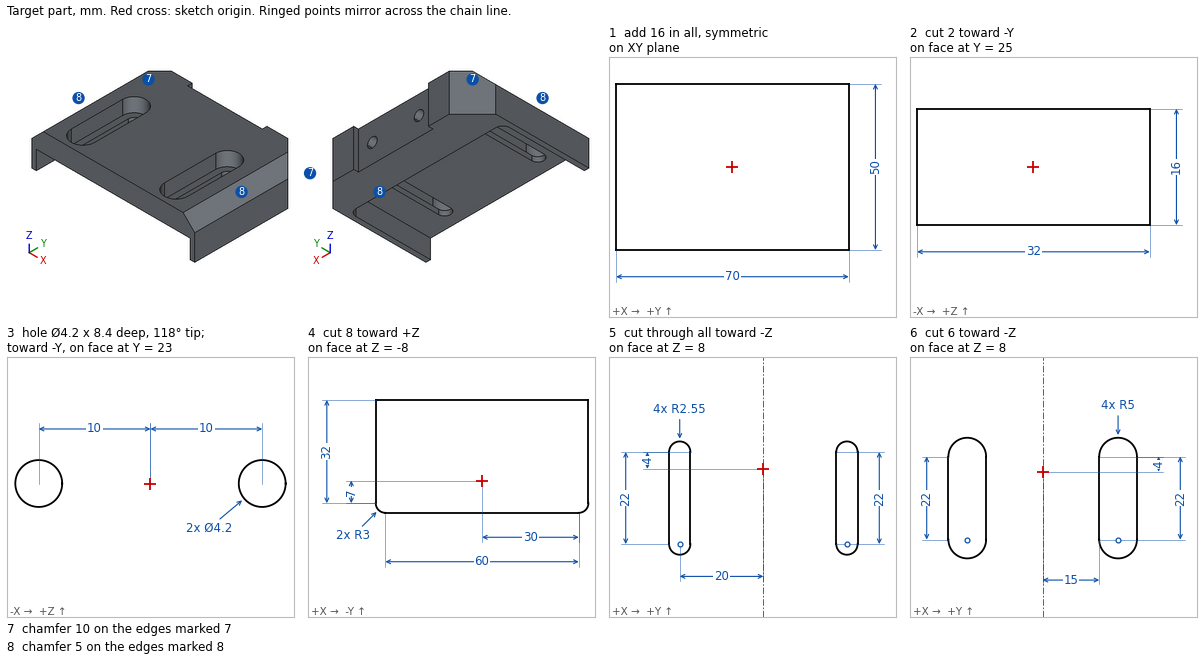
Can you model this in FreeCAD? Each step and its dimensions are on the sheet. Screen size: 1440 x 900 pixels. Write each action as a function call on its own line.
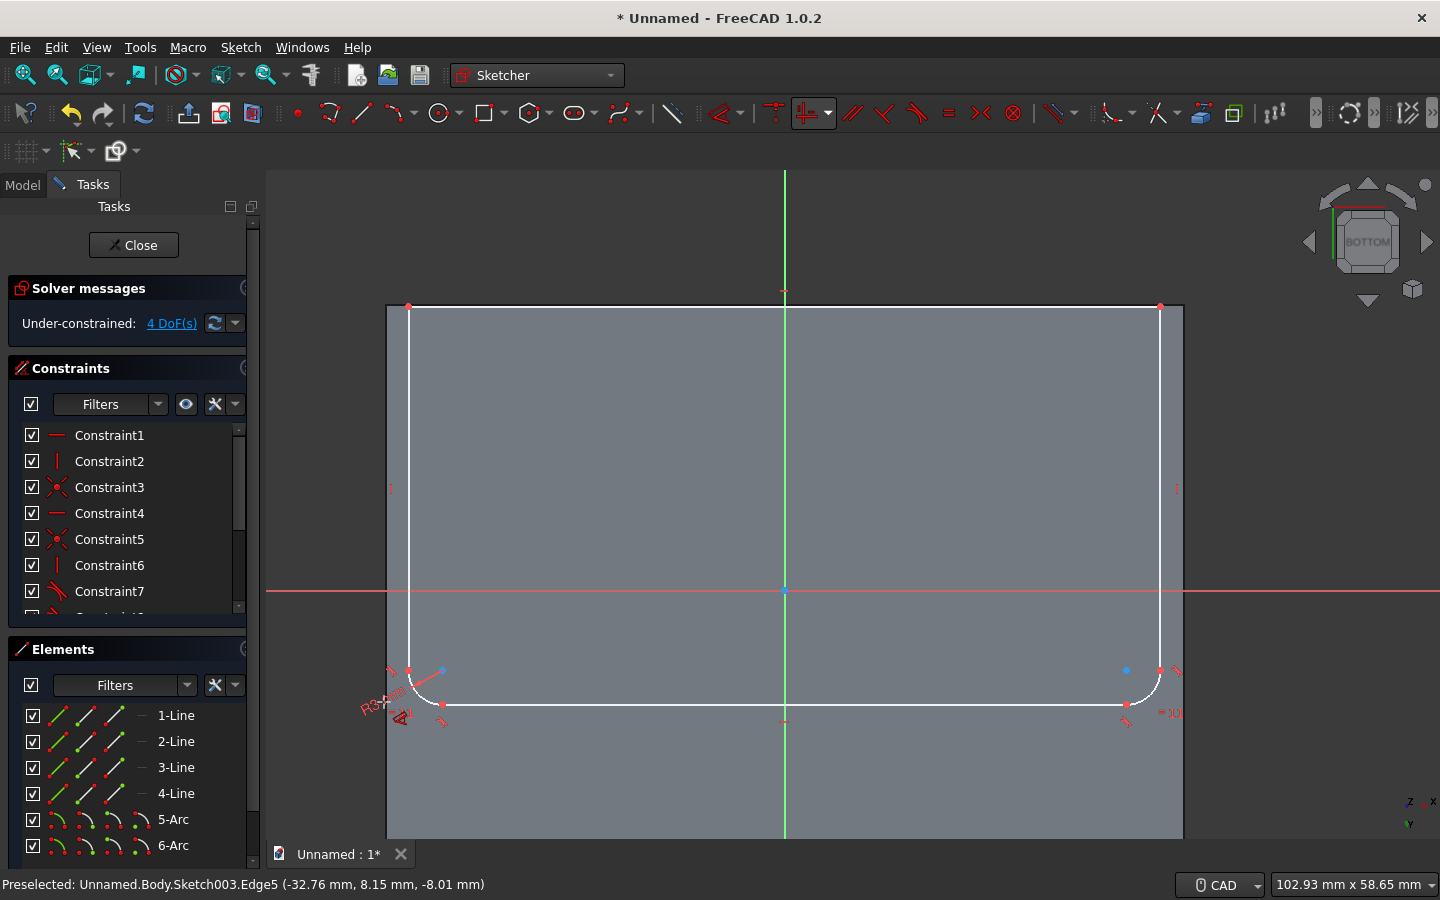
click(921, 705)
click(627, 739)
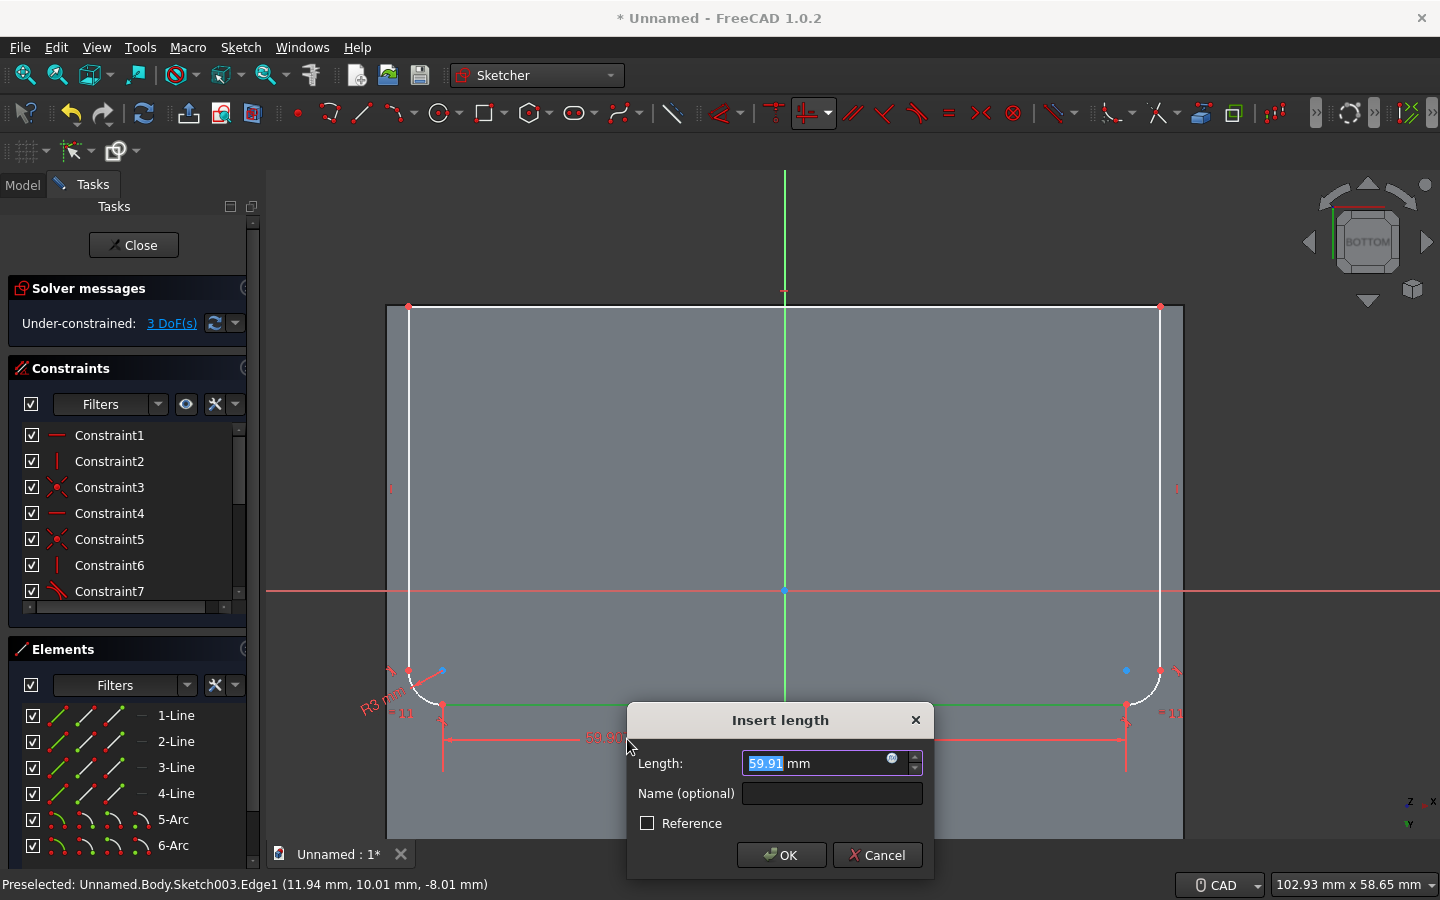
text(60)
key(Return)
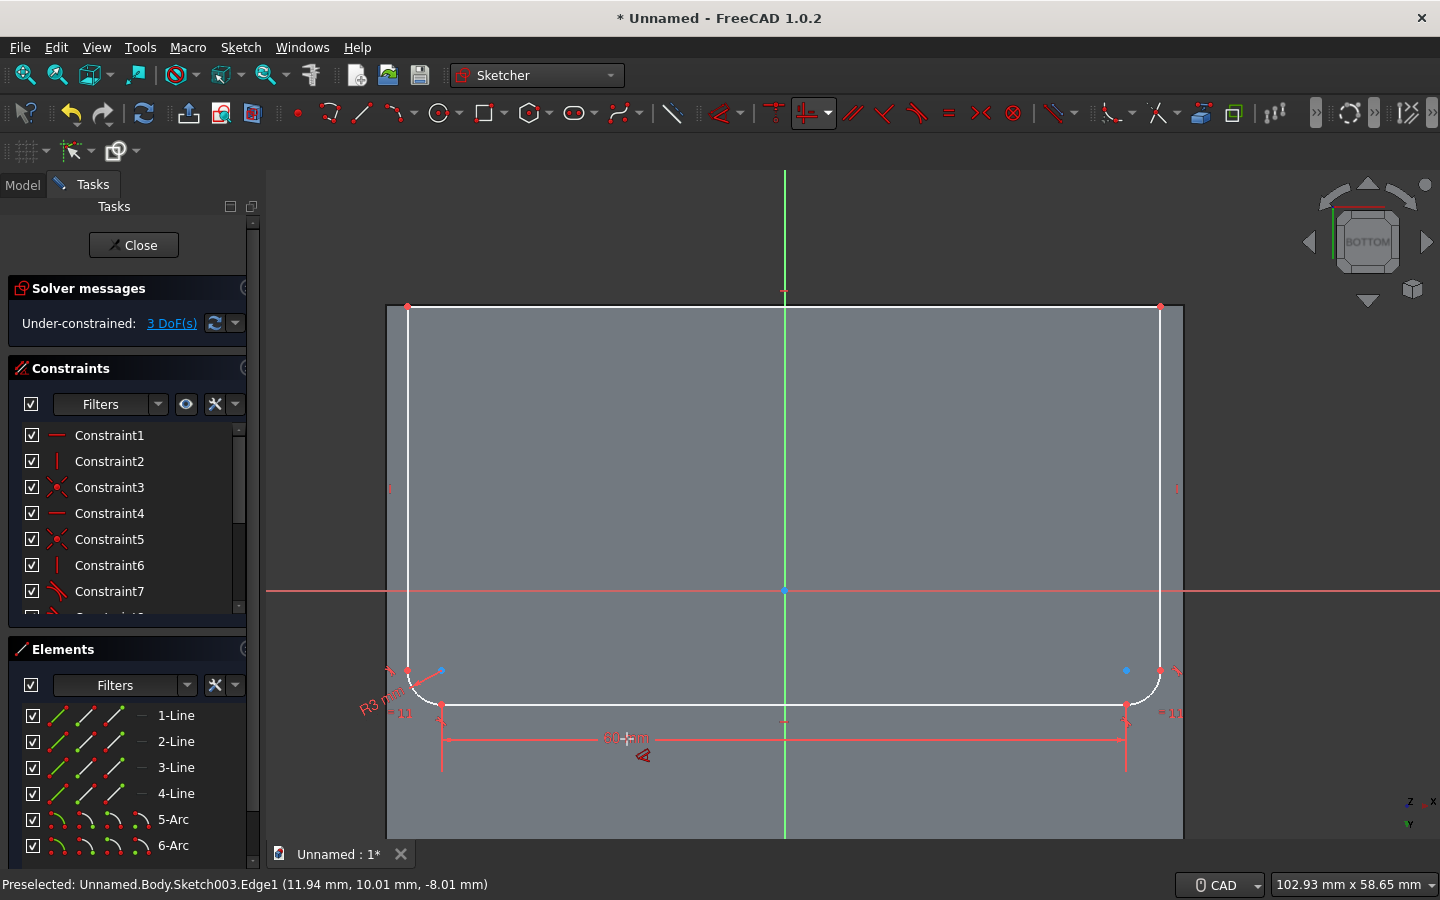
click(408, 561)
click(374, 489)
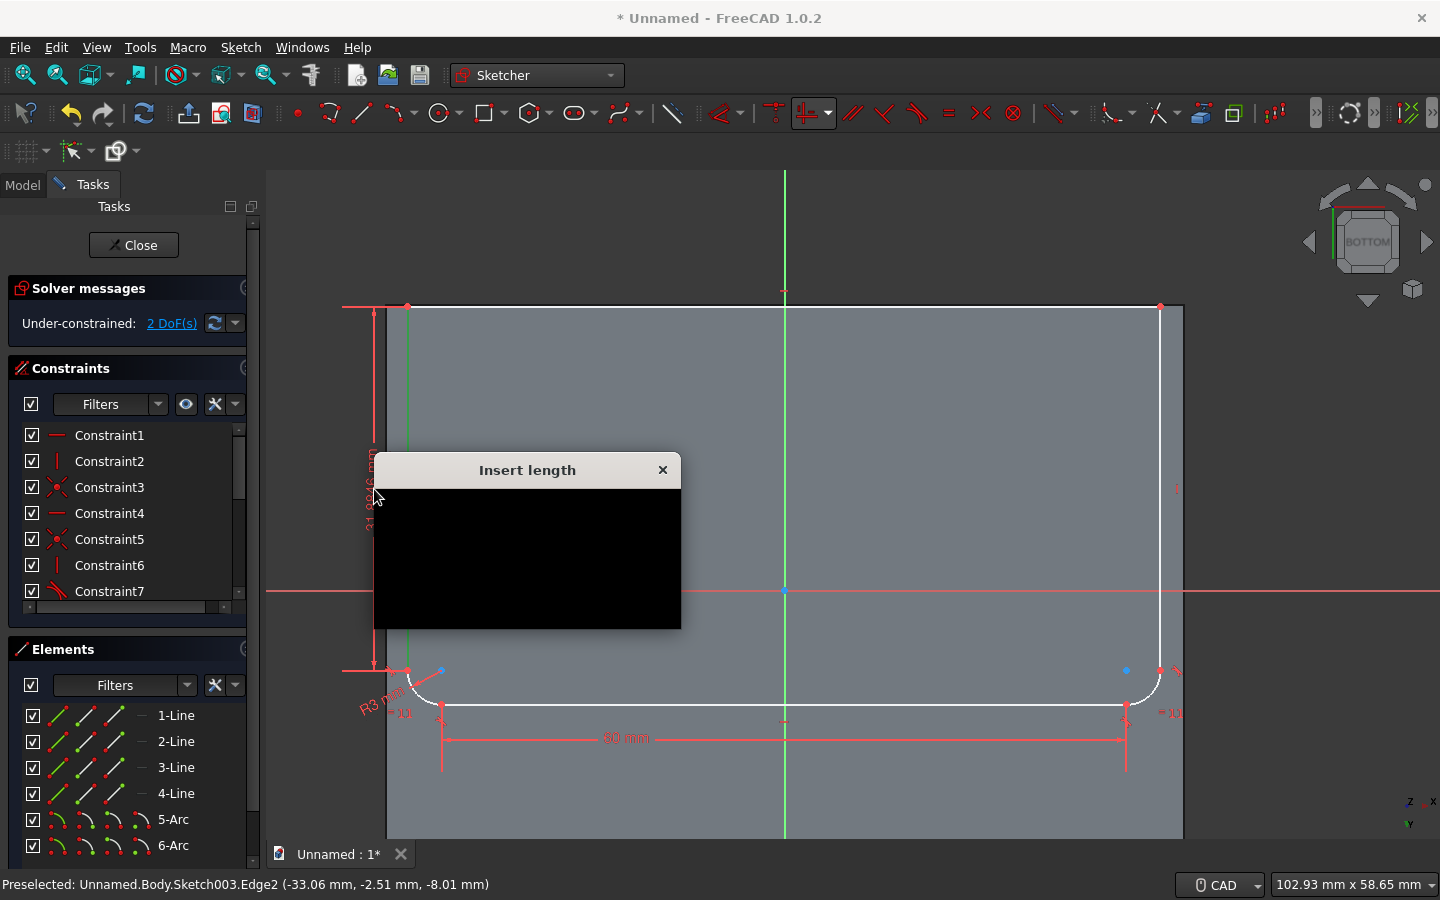
text(32)
key(Return)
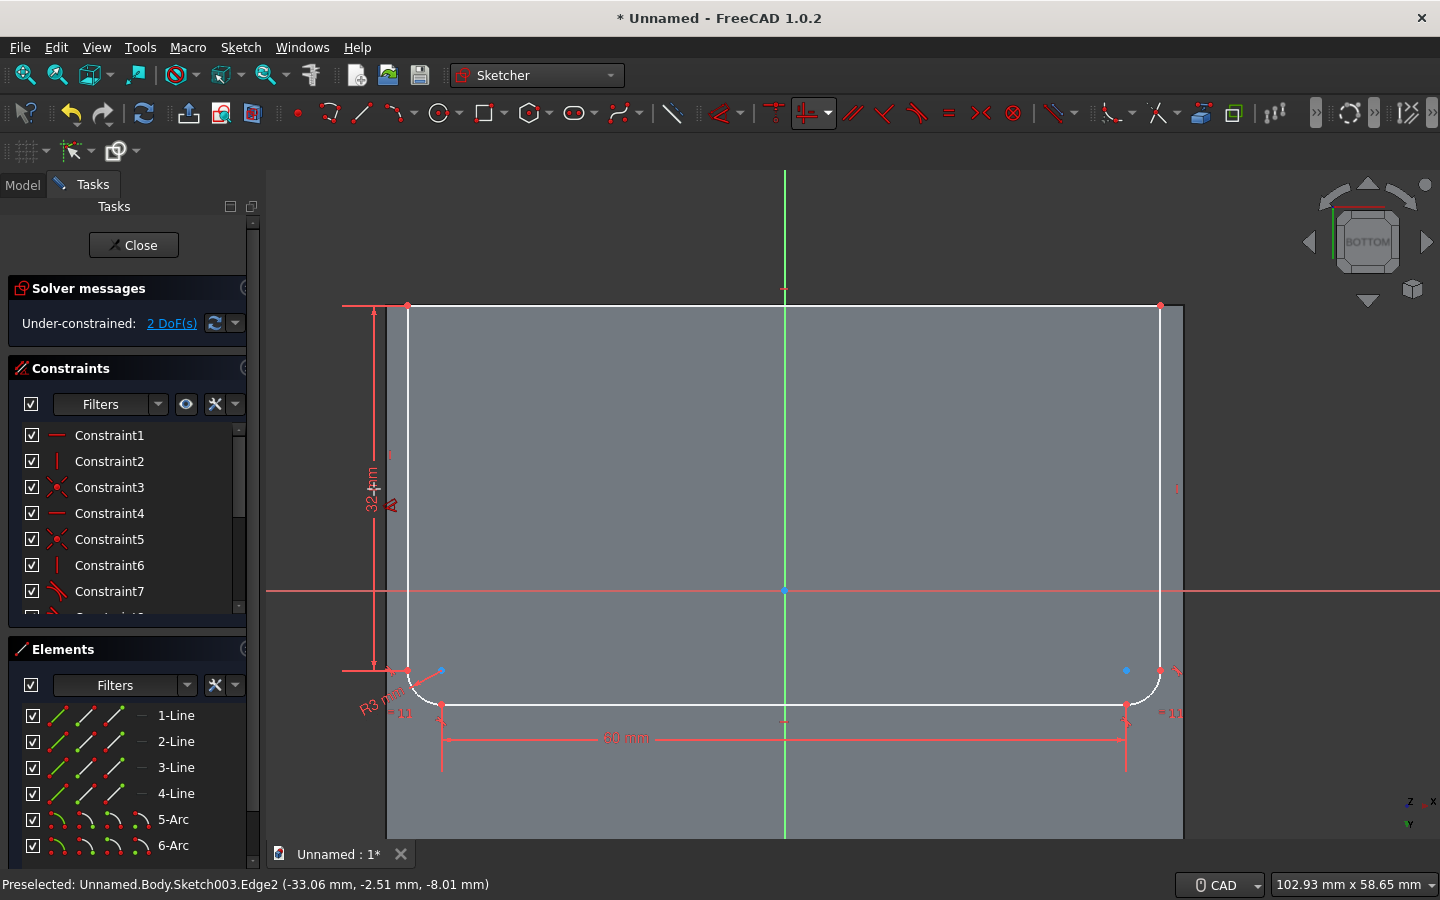
click(408, 671)
click(374, 631)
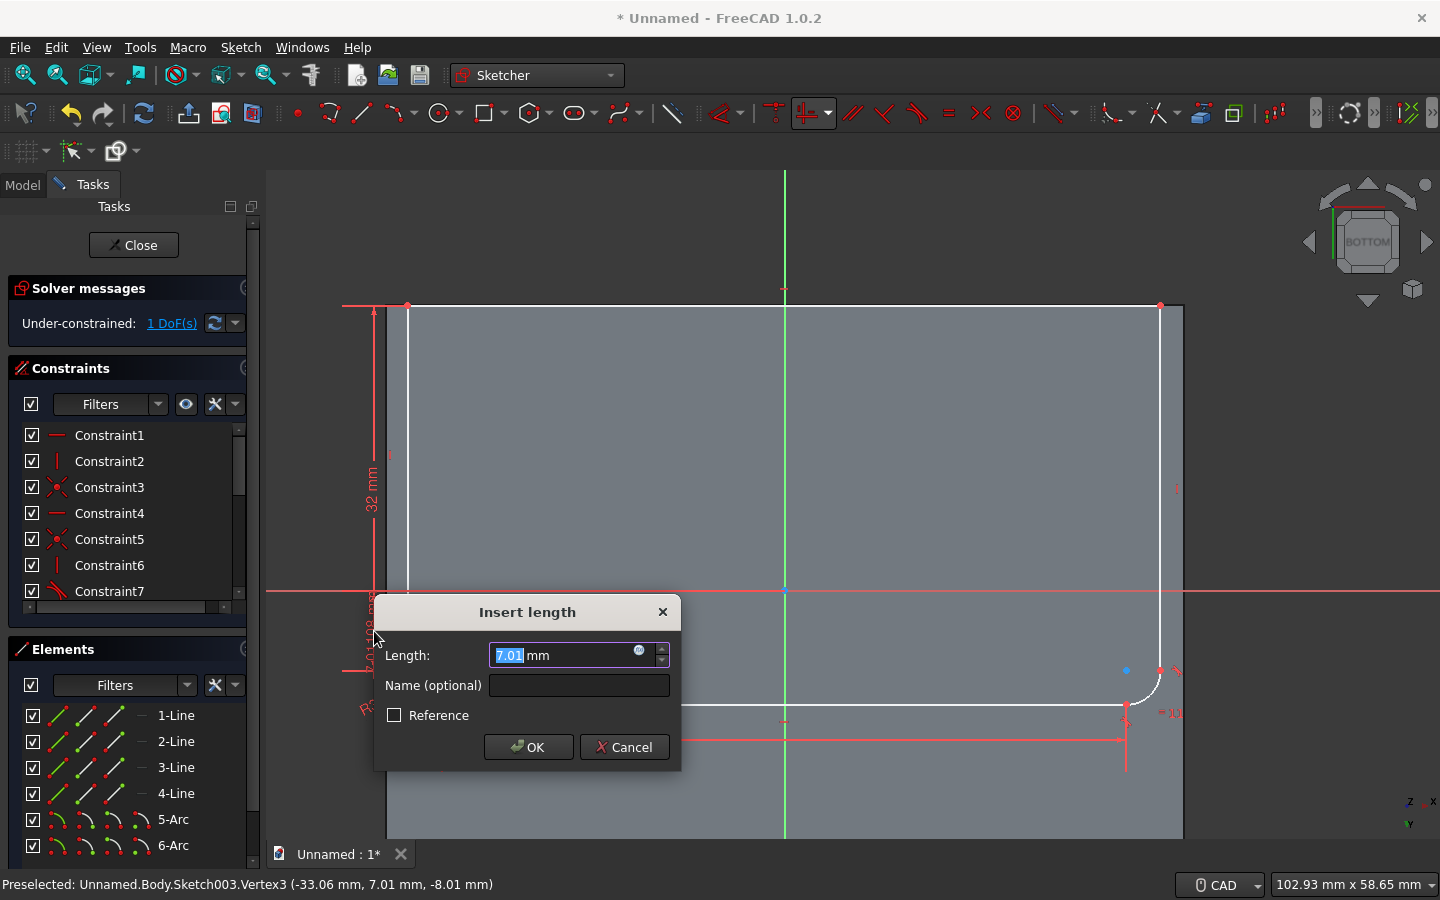
text(7)
key(Return)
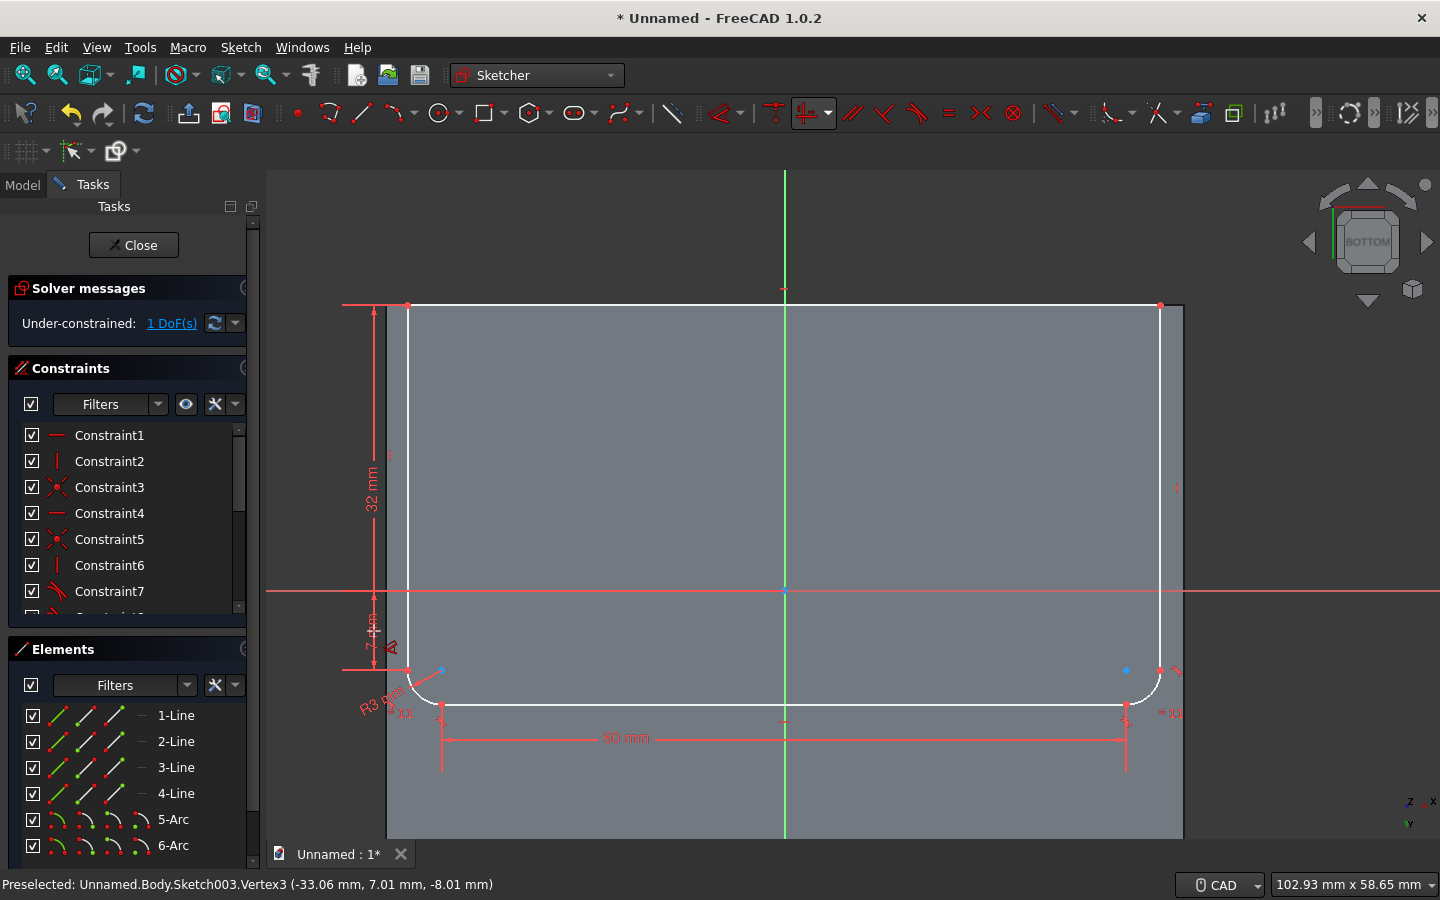
click(1126, 705)
click(956, 739)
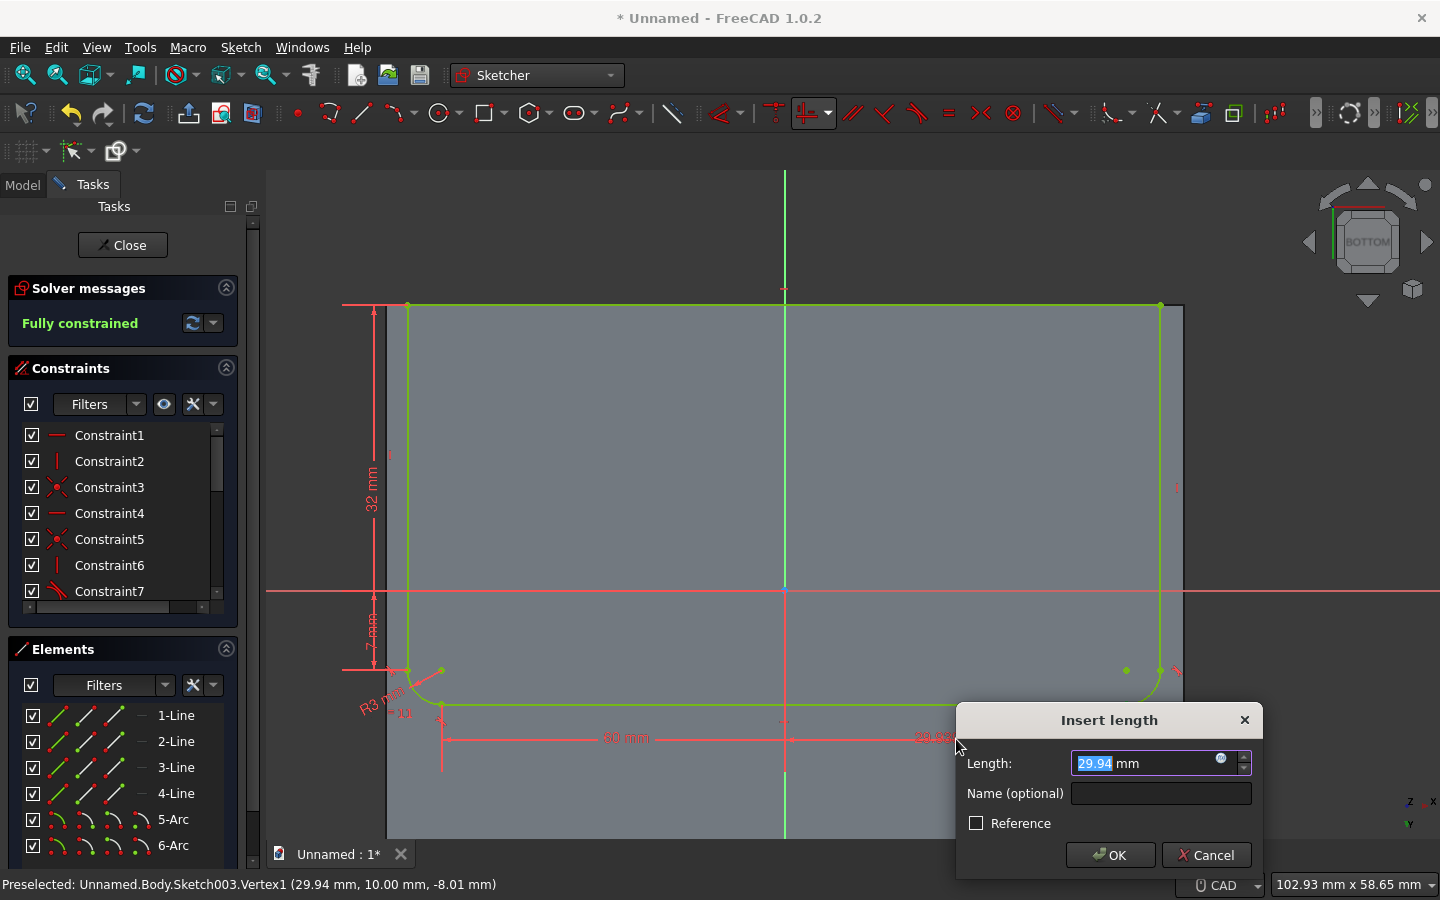
text(30)
key(Return)
key(Escape)